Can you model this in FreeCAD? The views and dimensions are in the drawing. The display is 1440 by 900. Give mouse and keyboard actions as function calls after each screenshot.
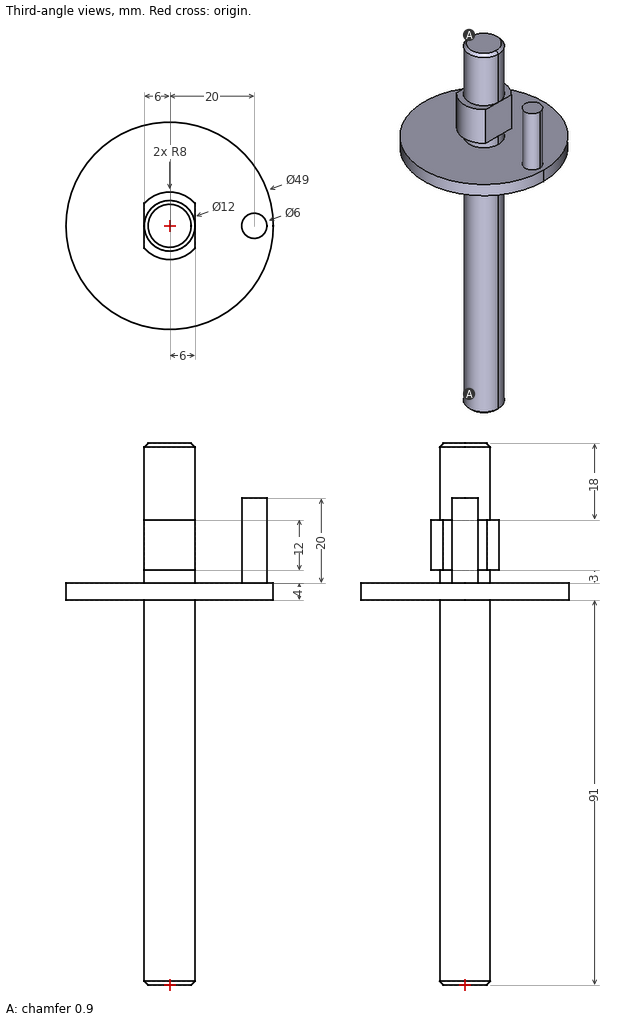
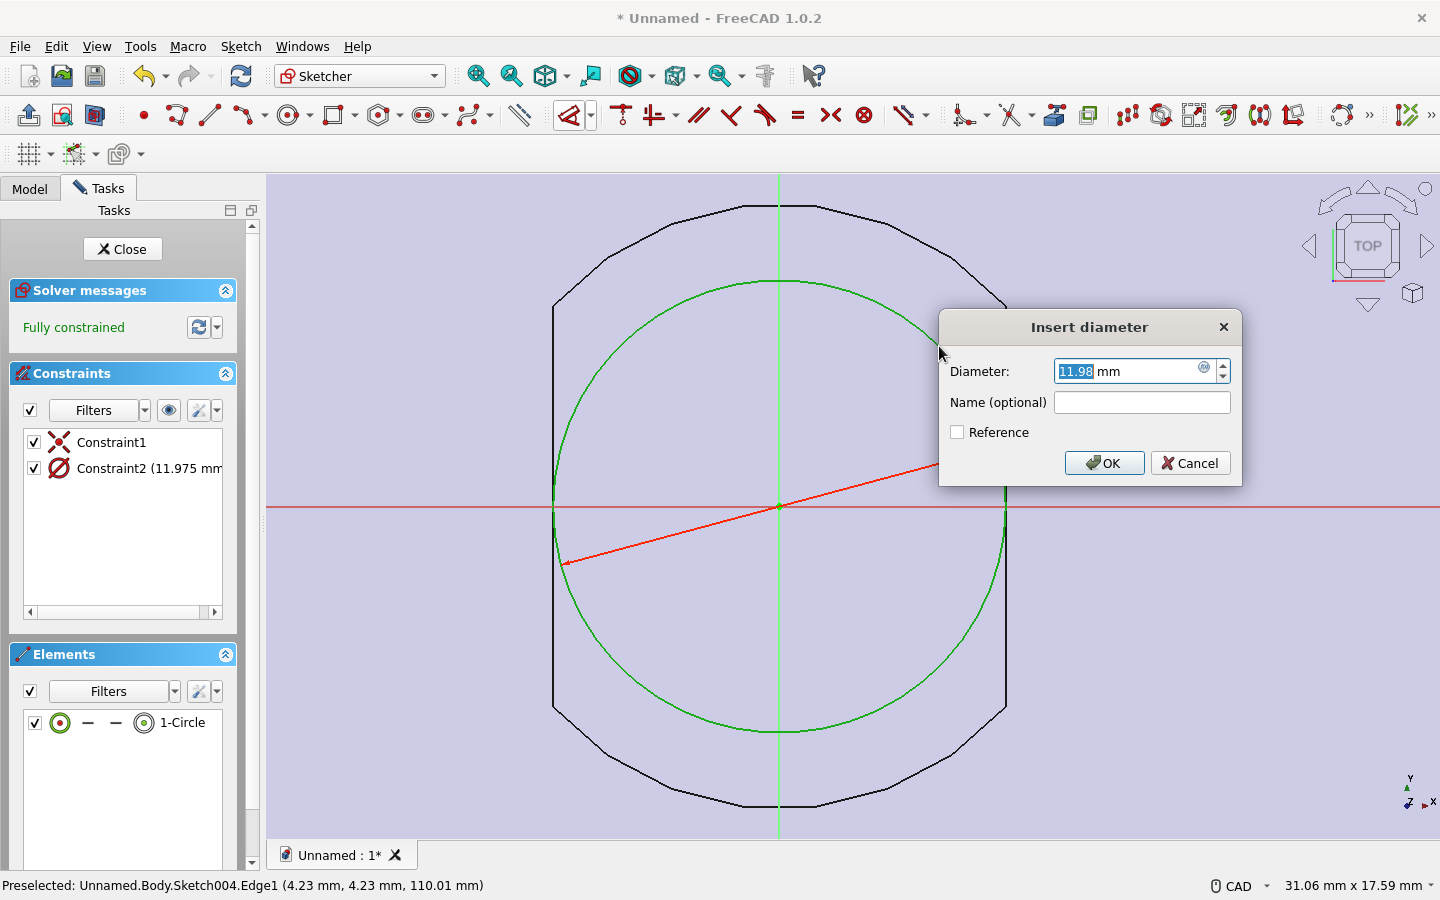
text(12)
key(Return)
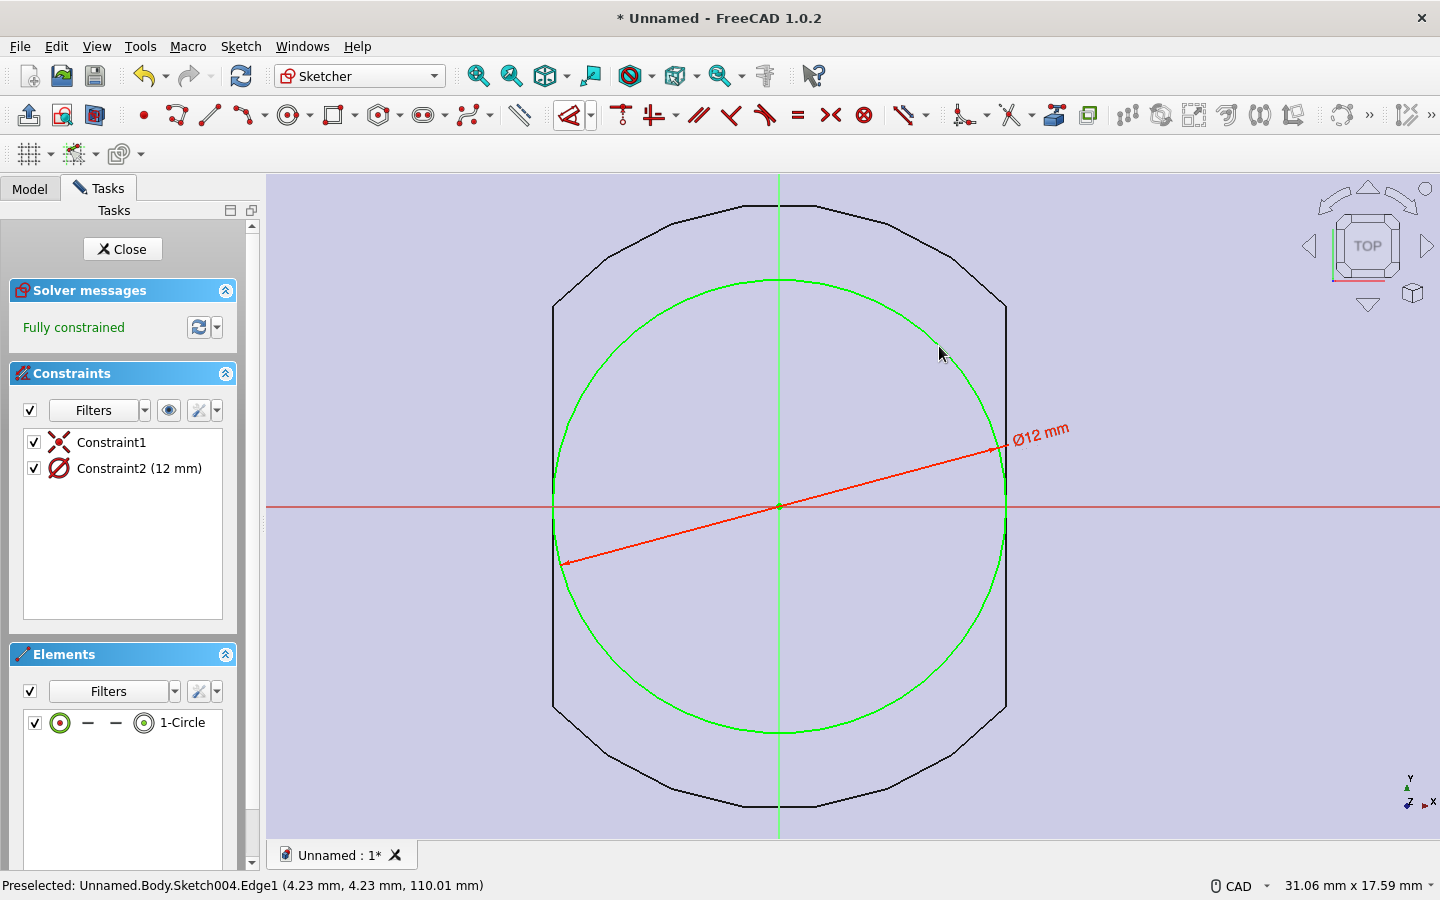
click(123, 249)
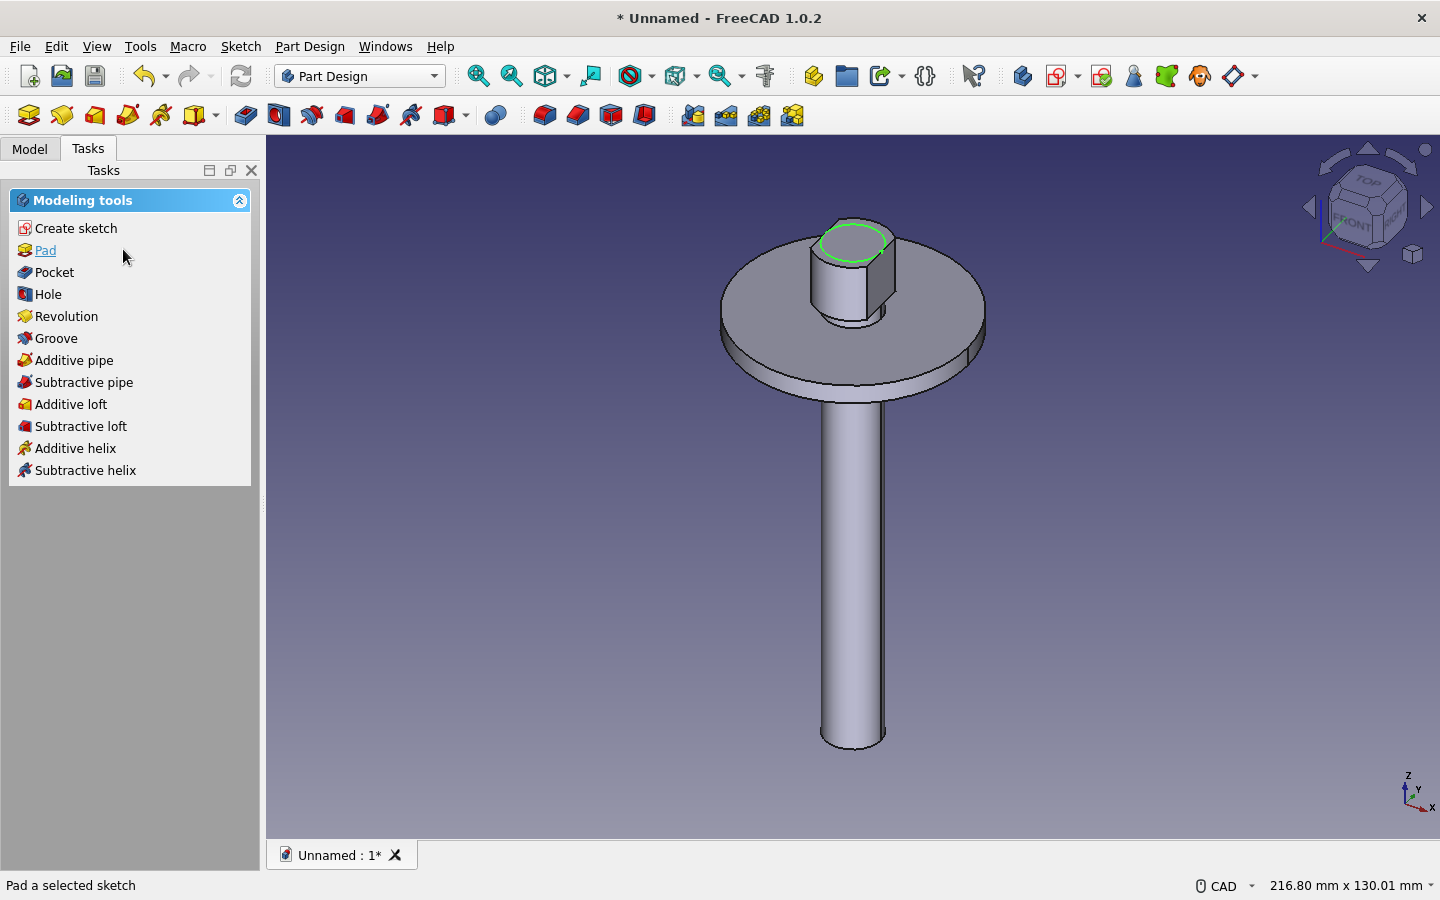
click(29, 116)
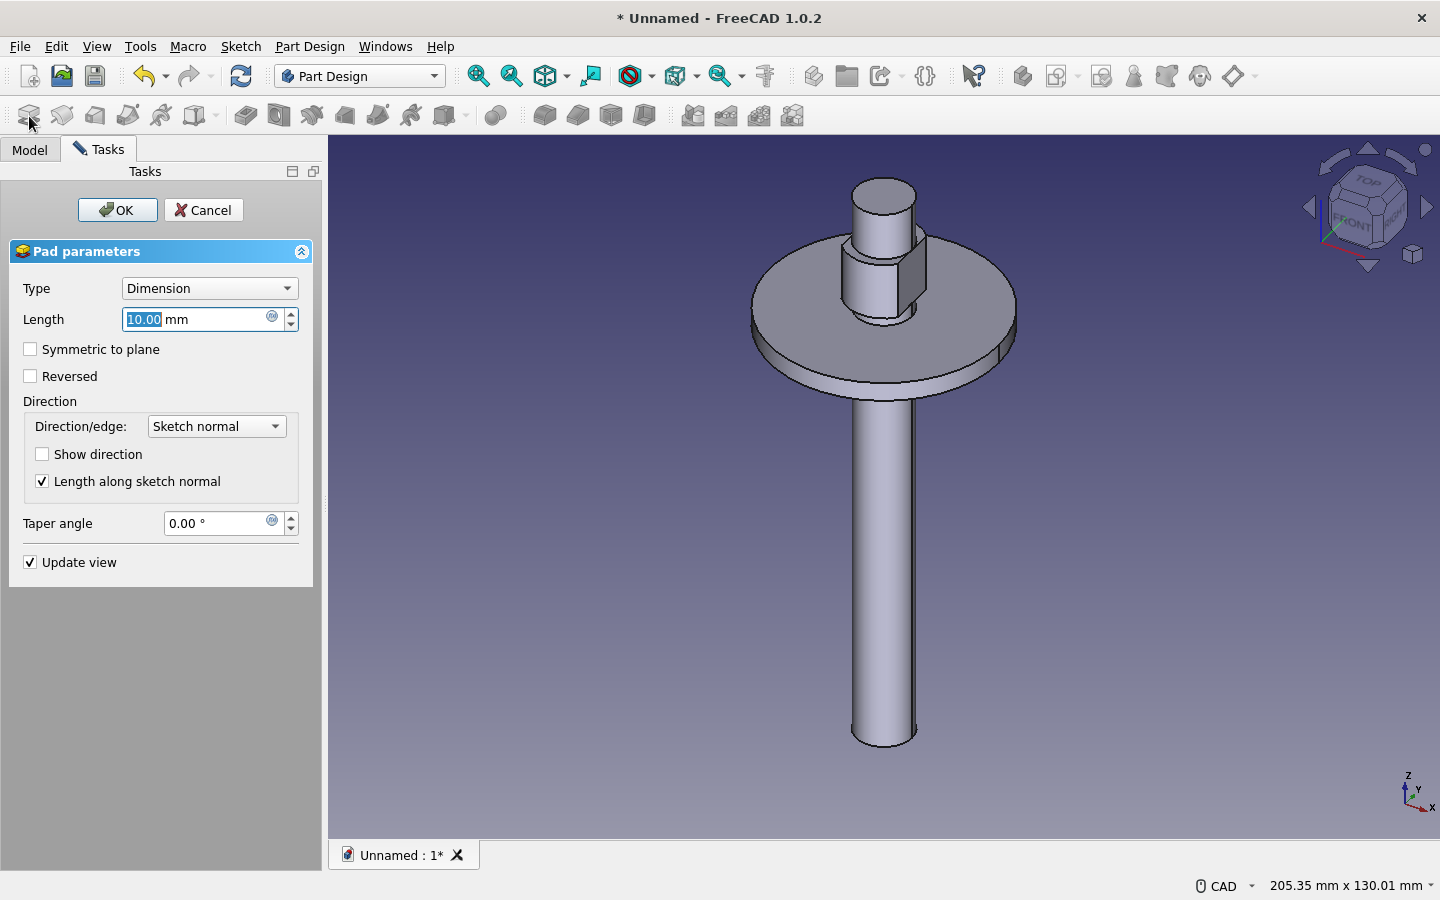
text(18)
key(Tab)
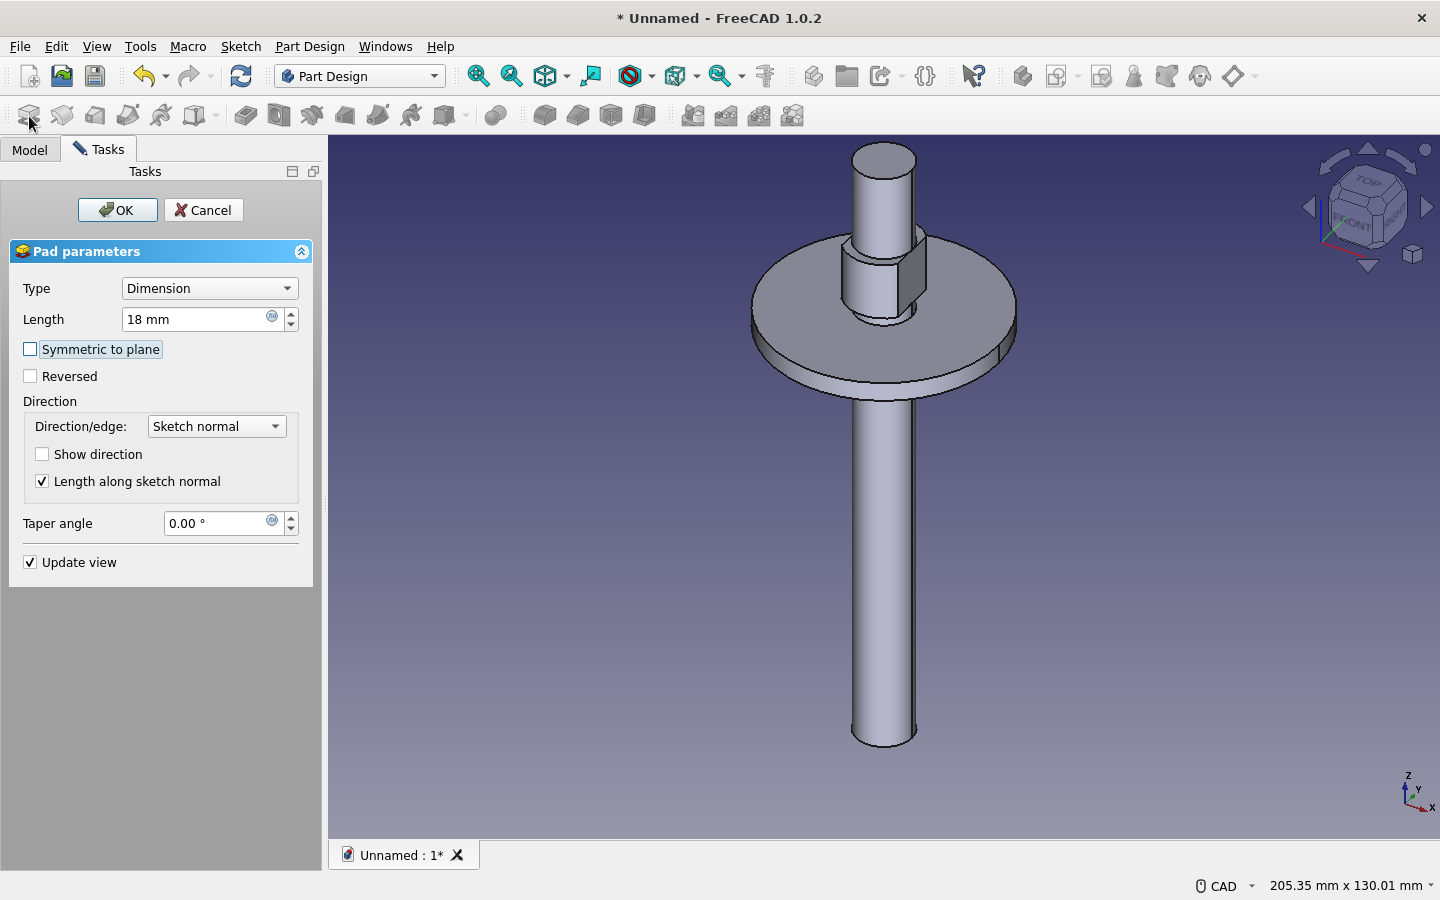
click(118, 210)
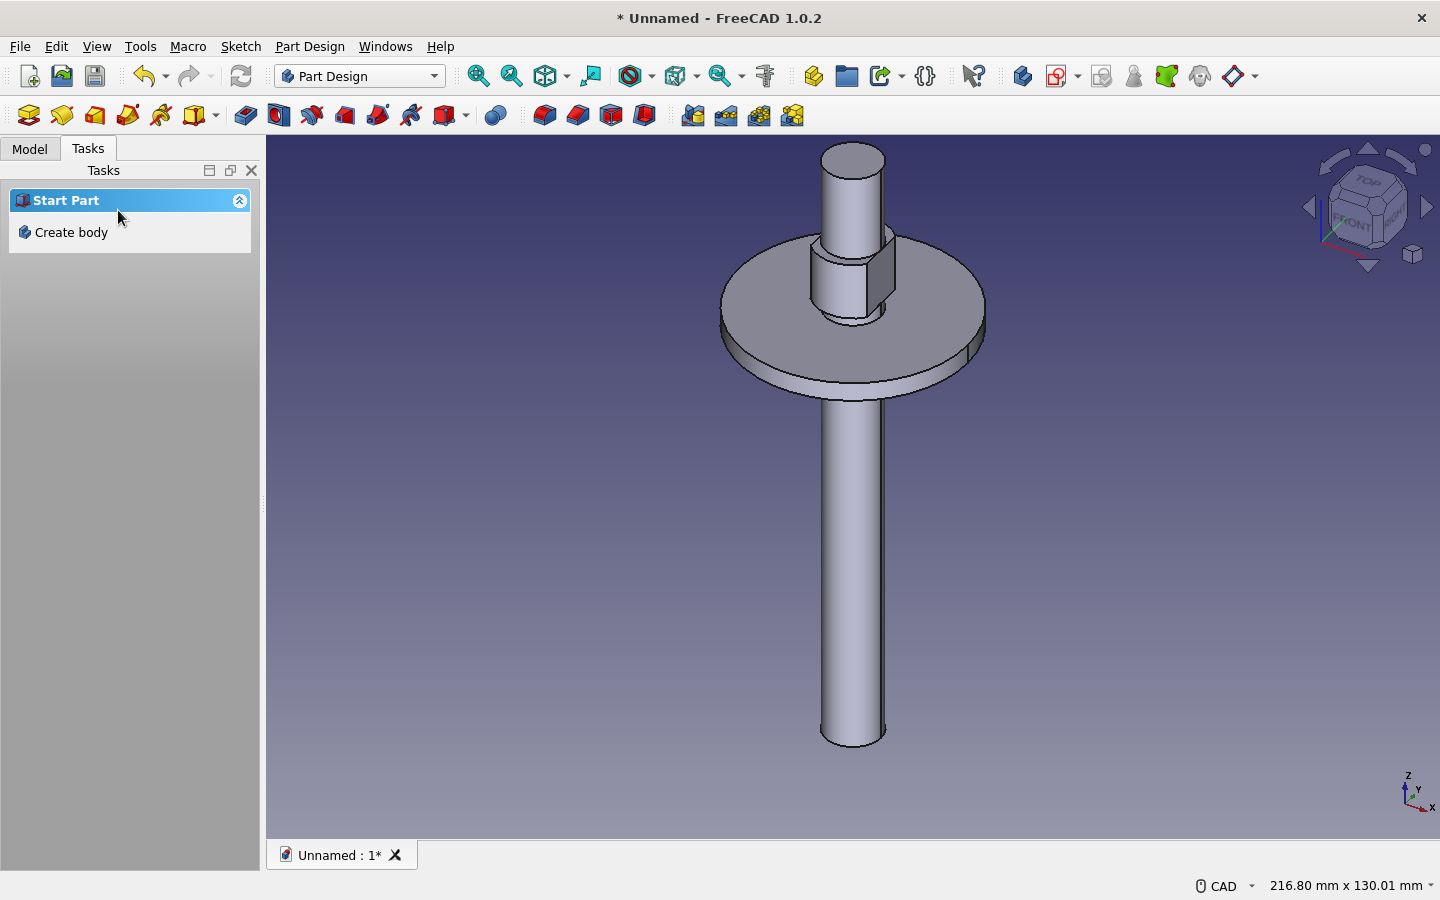
key(v)
key(f)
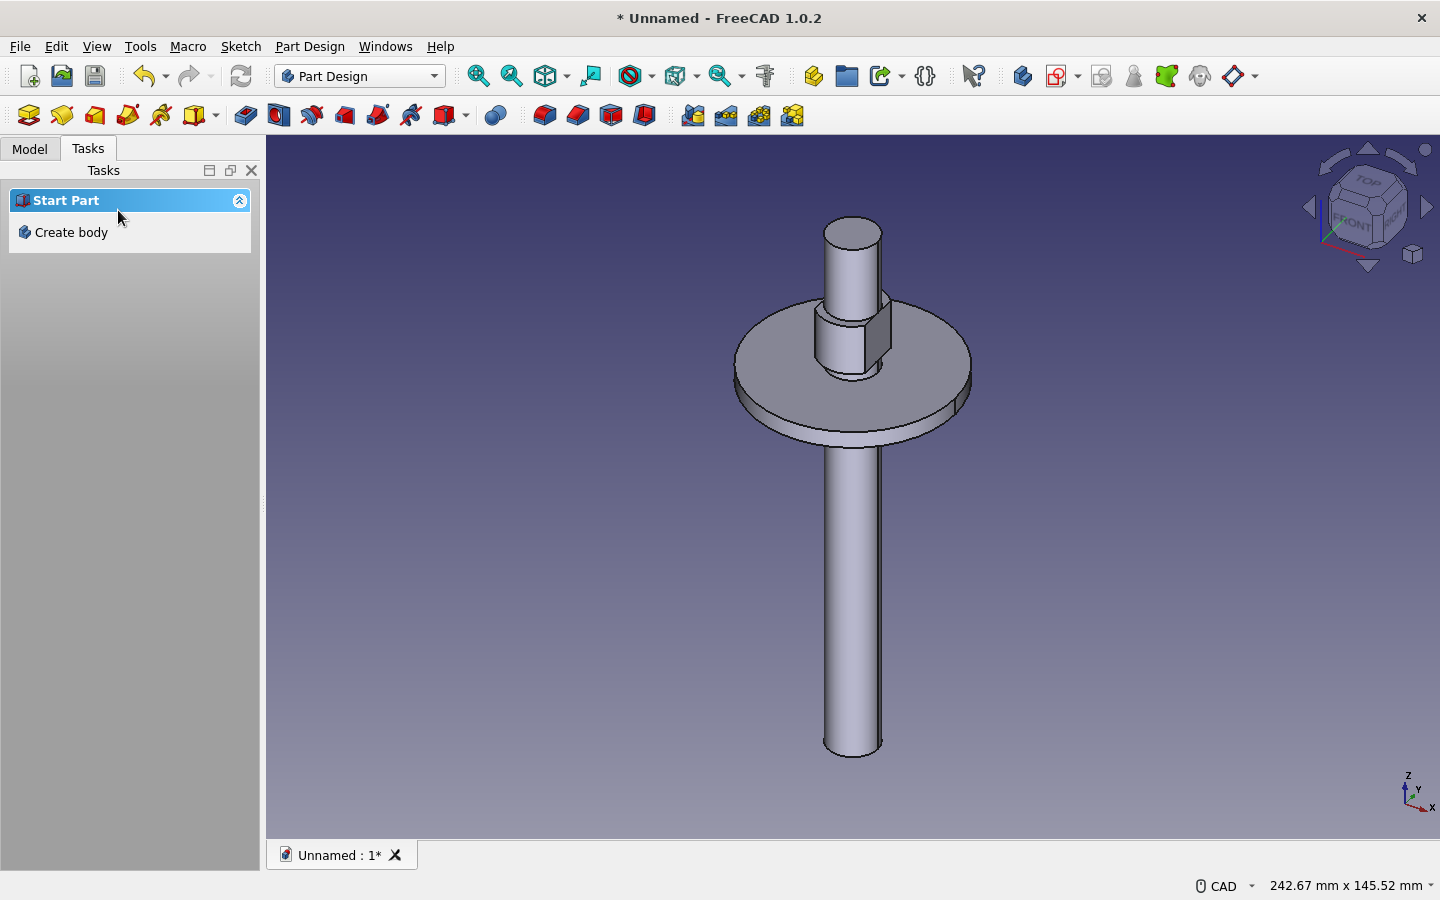
click(831, 751)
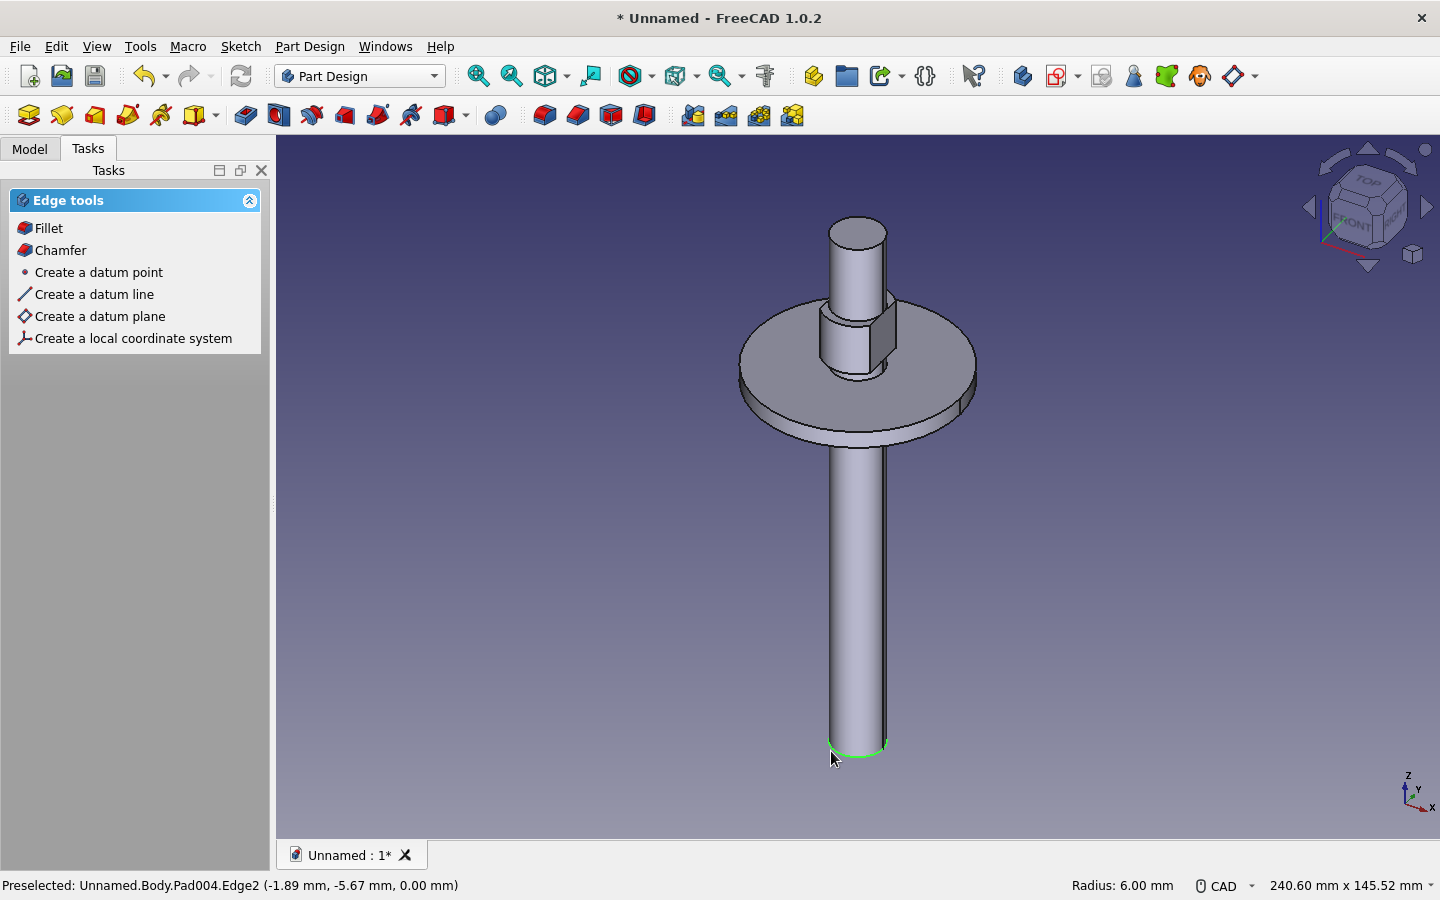
click(829, 234, ctrl)